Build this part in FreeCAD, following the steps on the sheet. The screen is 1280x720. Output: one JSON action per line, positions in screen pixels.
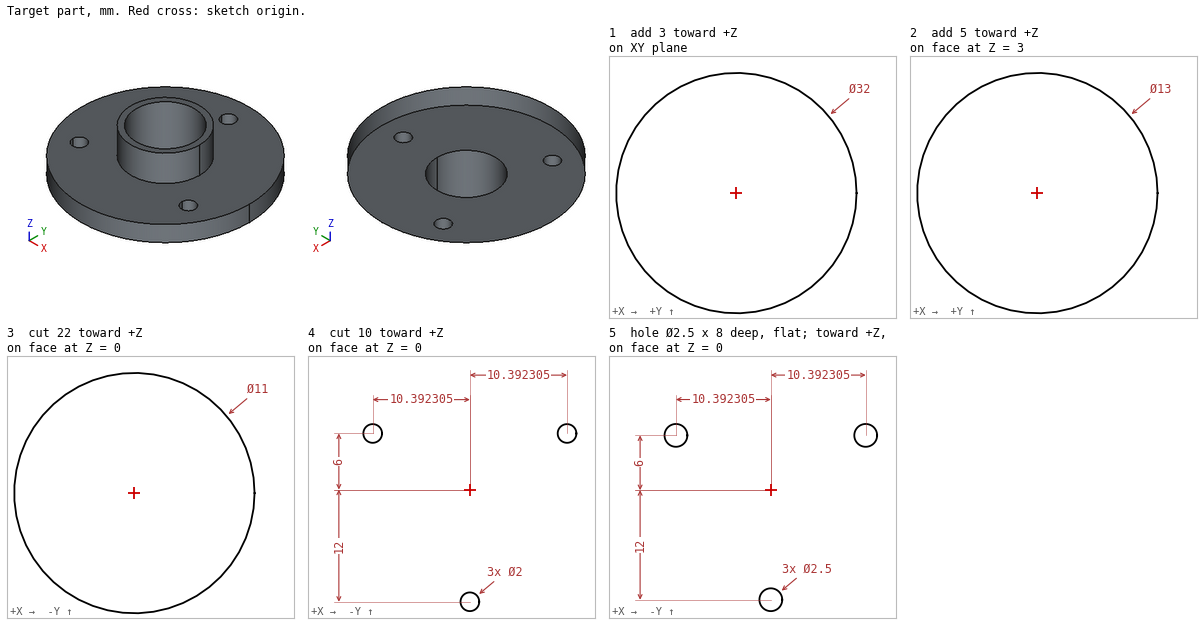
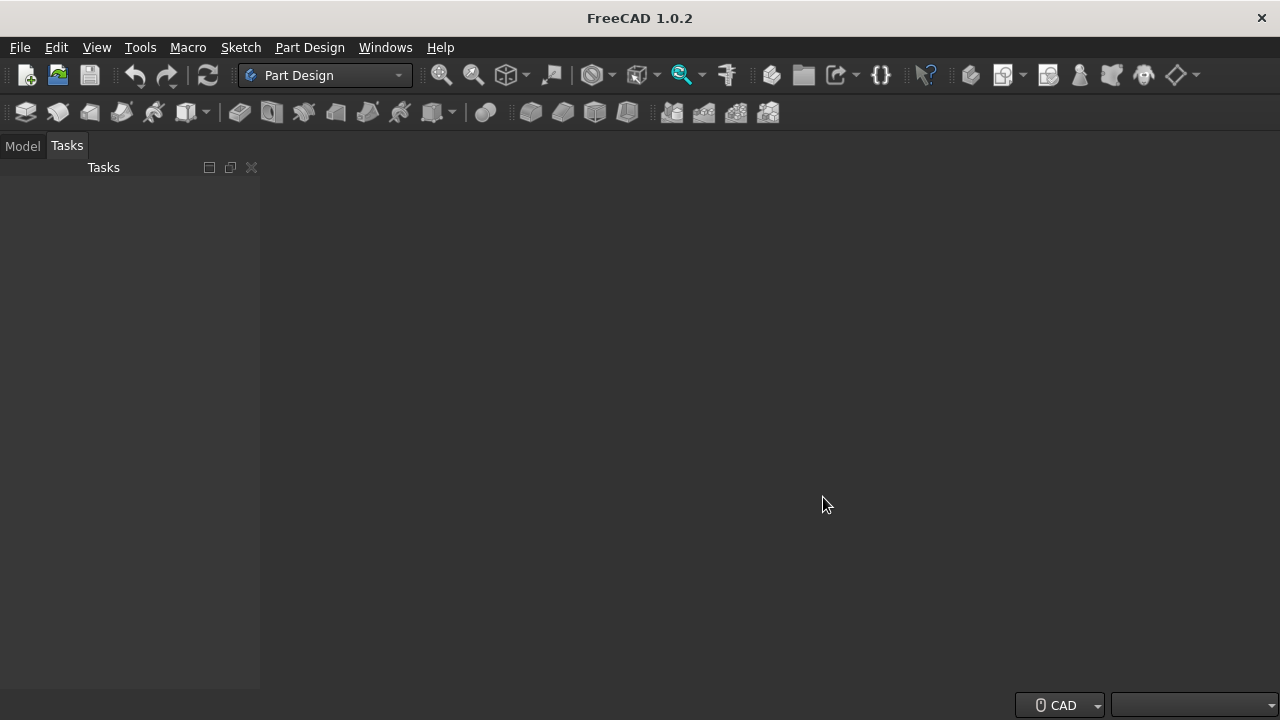
{"action": "left_click", "coordinate": [26, 76]}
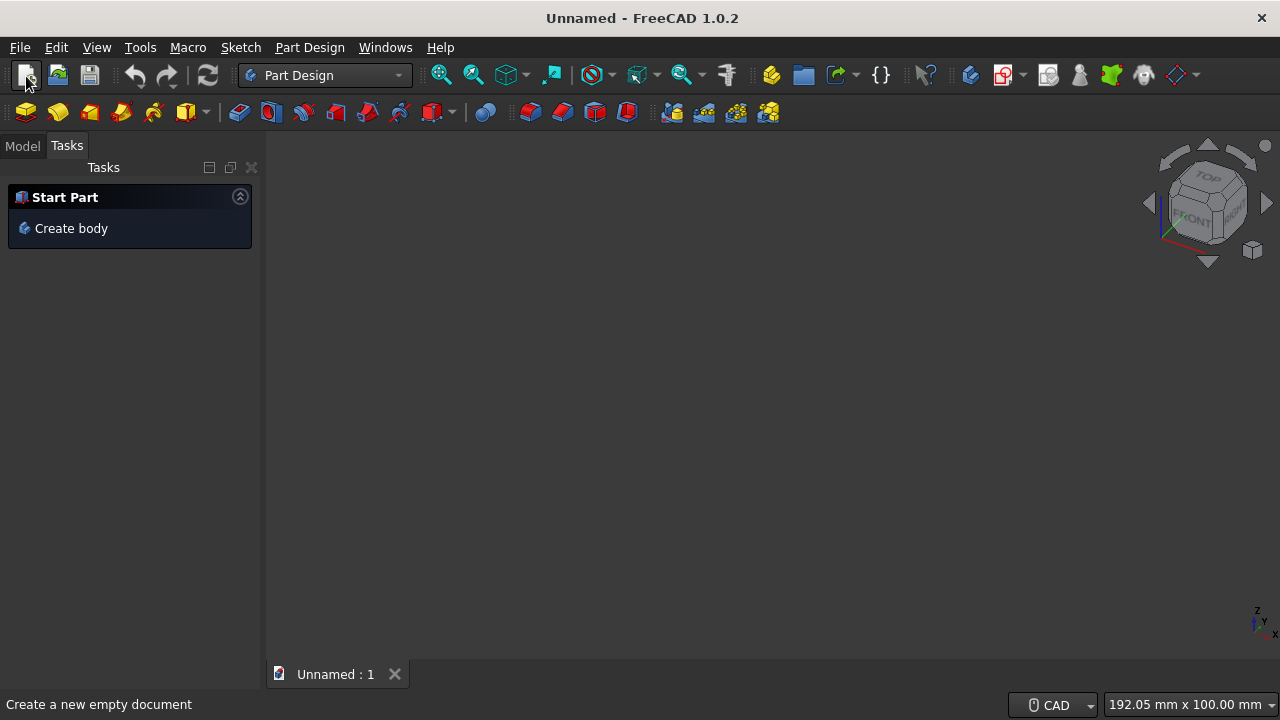
{"action": "left_click", "coordinate": [1004, 76]}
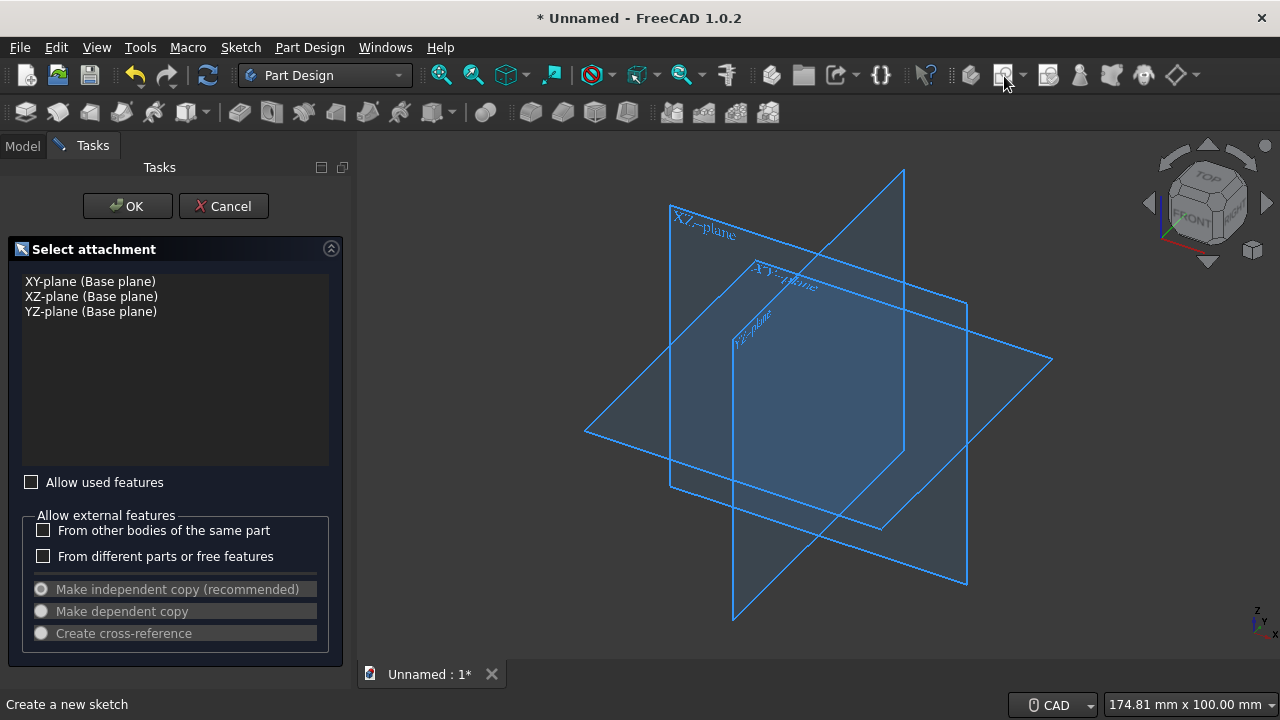
{"action": "left_click", "coordinate": [82, 282]}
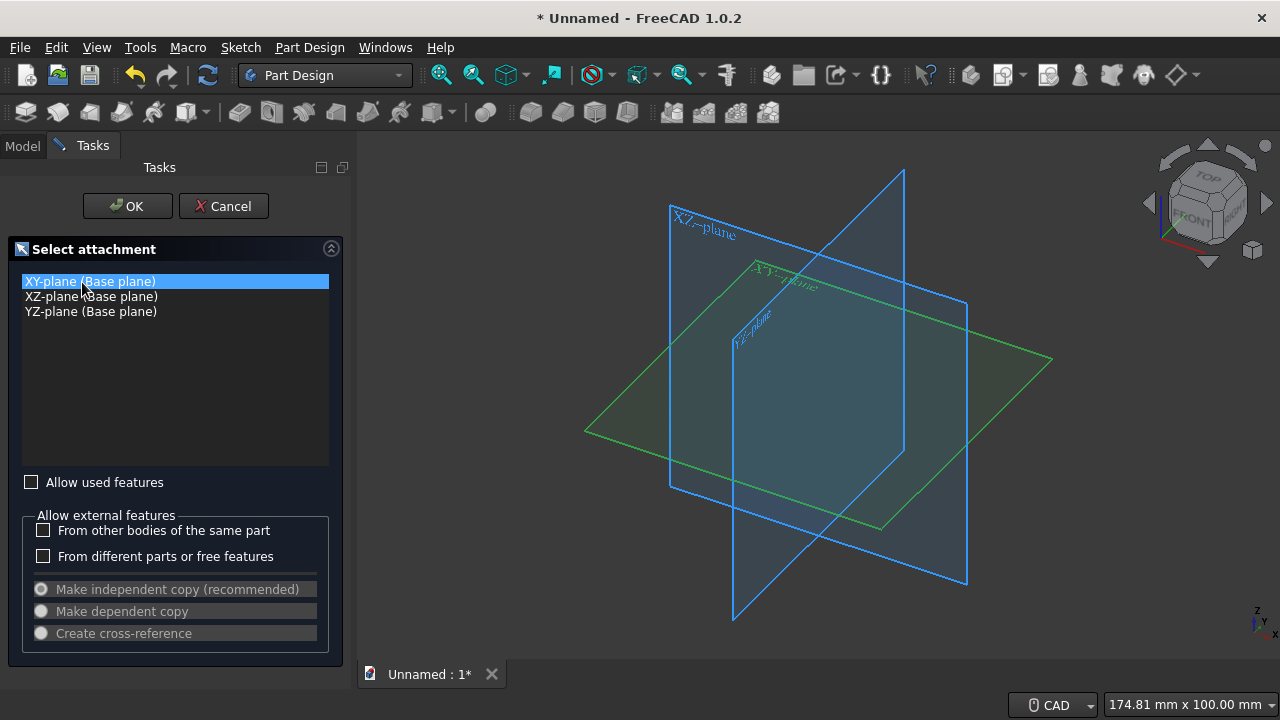
{"action": "left_click", "coordinate": [128, 206]}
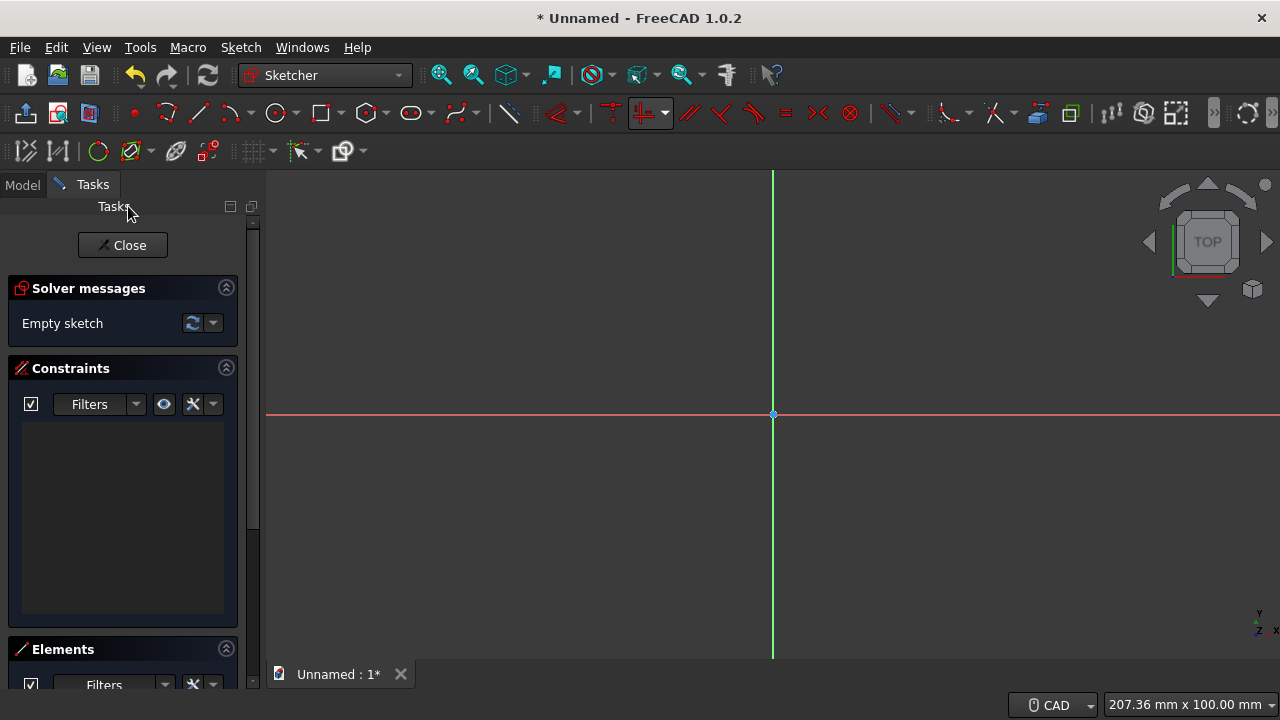
{"action": "scroll", "coordinate": [856, 415], "scroll_direction": "up", "scroll_amount": 3}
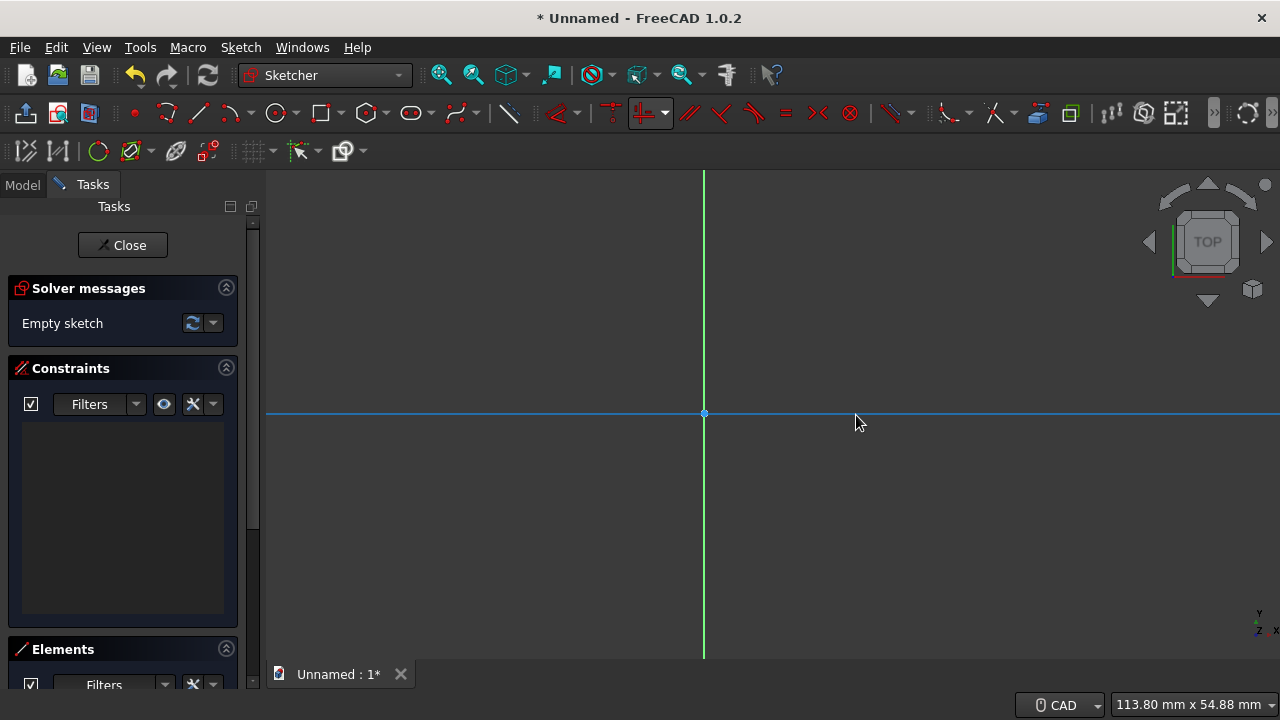
{"action": "left_click", "coordinate": [276, 114]}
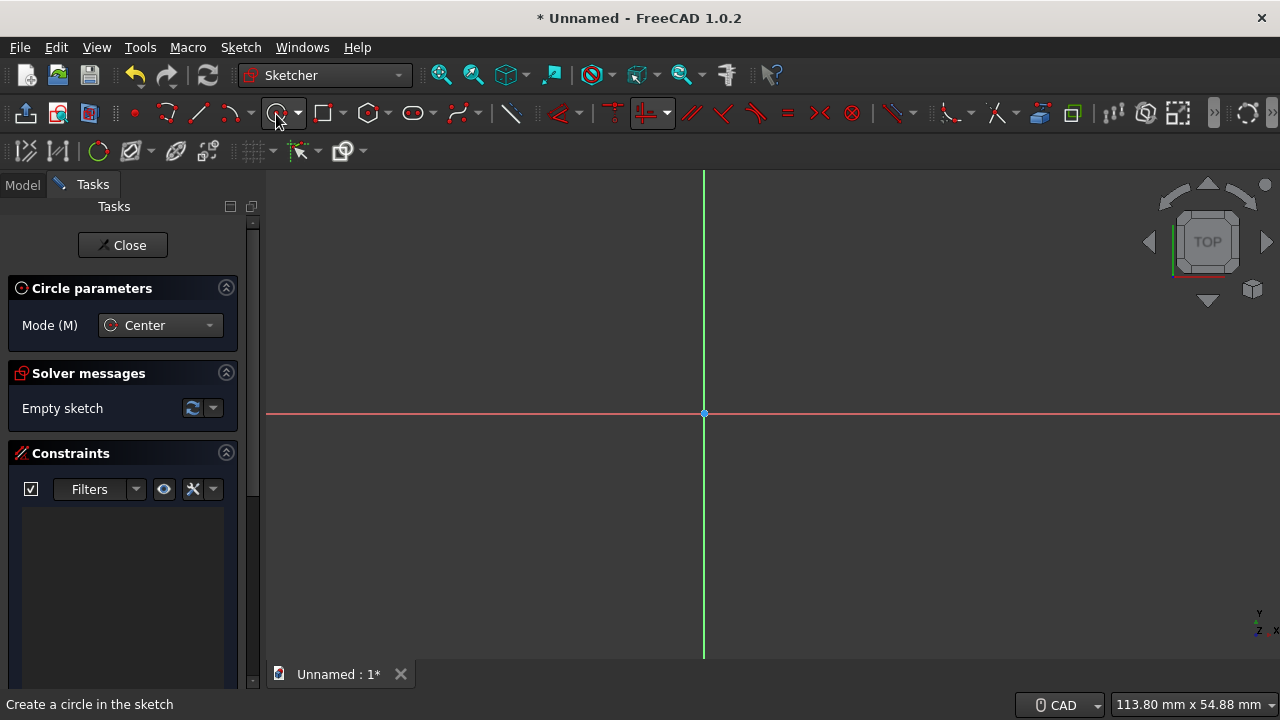
{"action": "left_click", "coordinate": [704, 414]}
{"action": "mouse_move", "coordinate": [805, 313]}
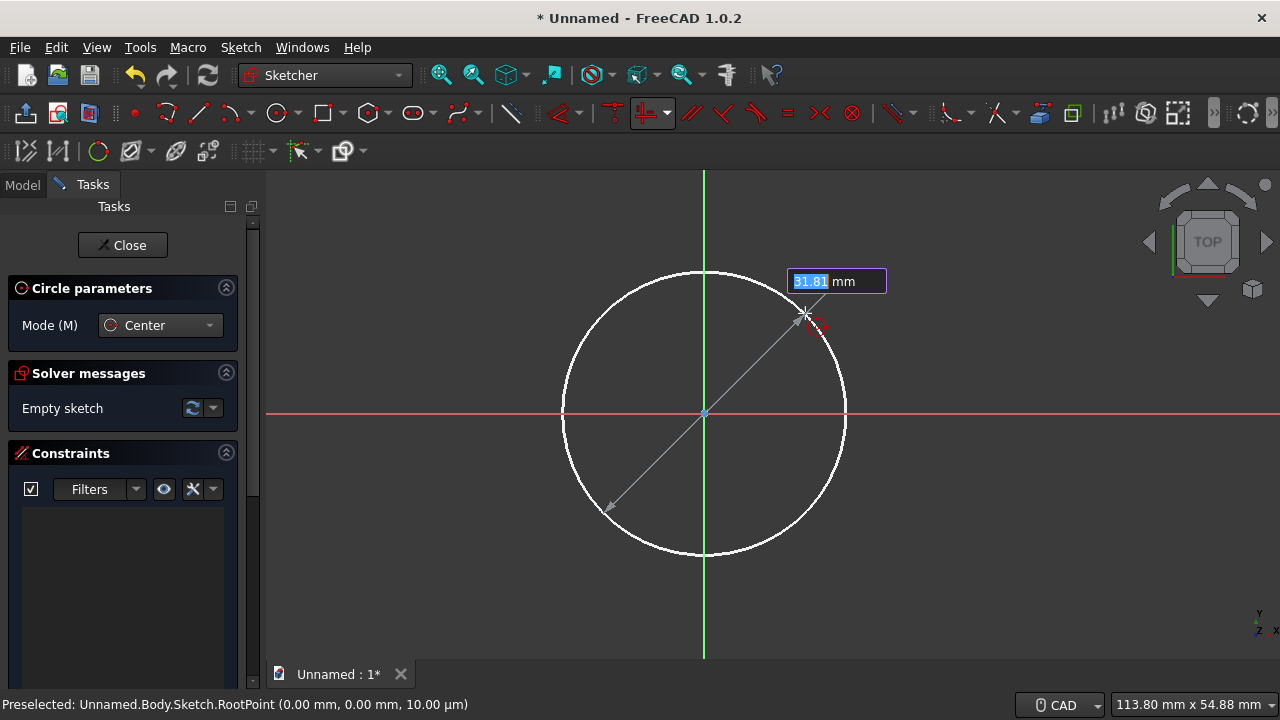
{"action": "type", "text": "32"}
{"action": "key", "text": "Return"}
{"action": "key", "text": "Escape"}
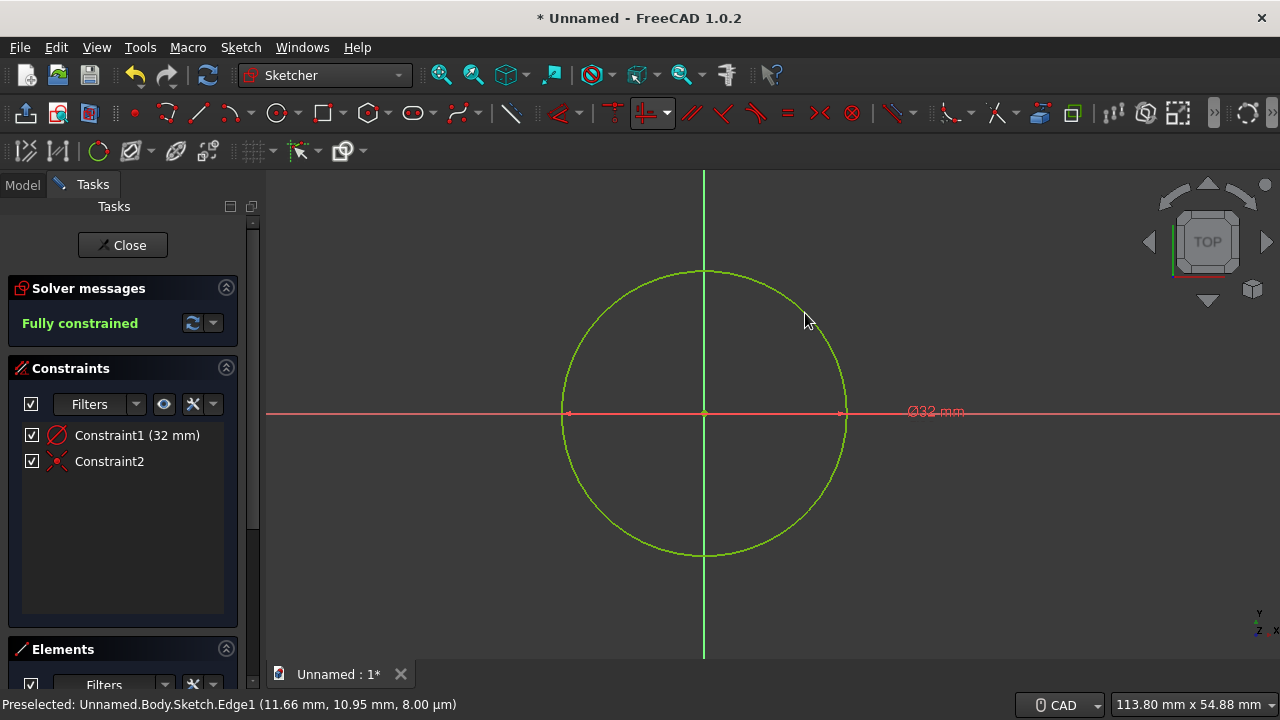
{"action": "left_click", "coordinate": [123, 245]}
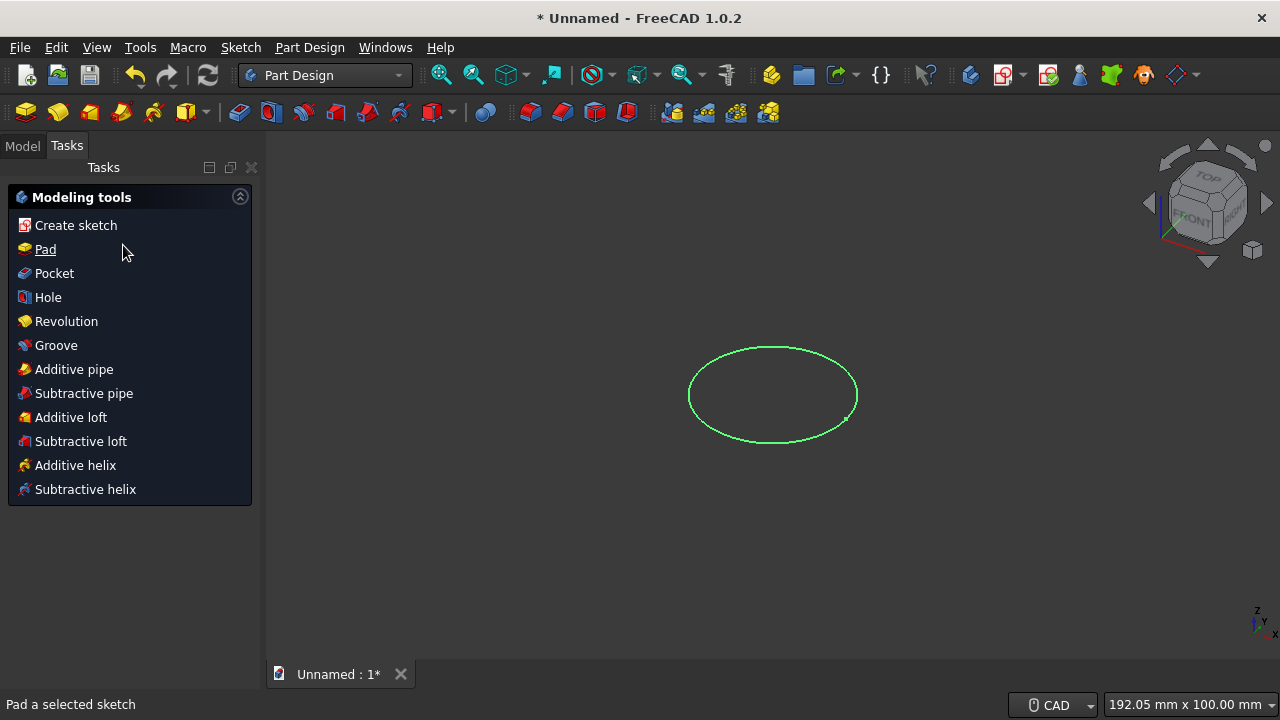
{"action": "left_click", "coordinate": [26, 112]}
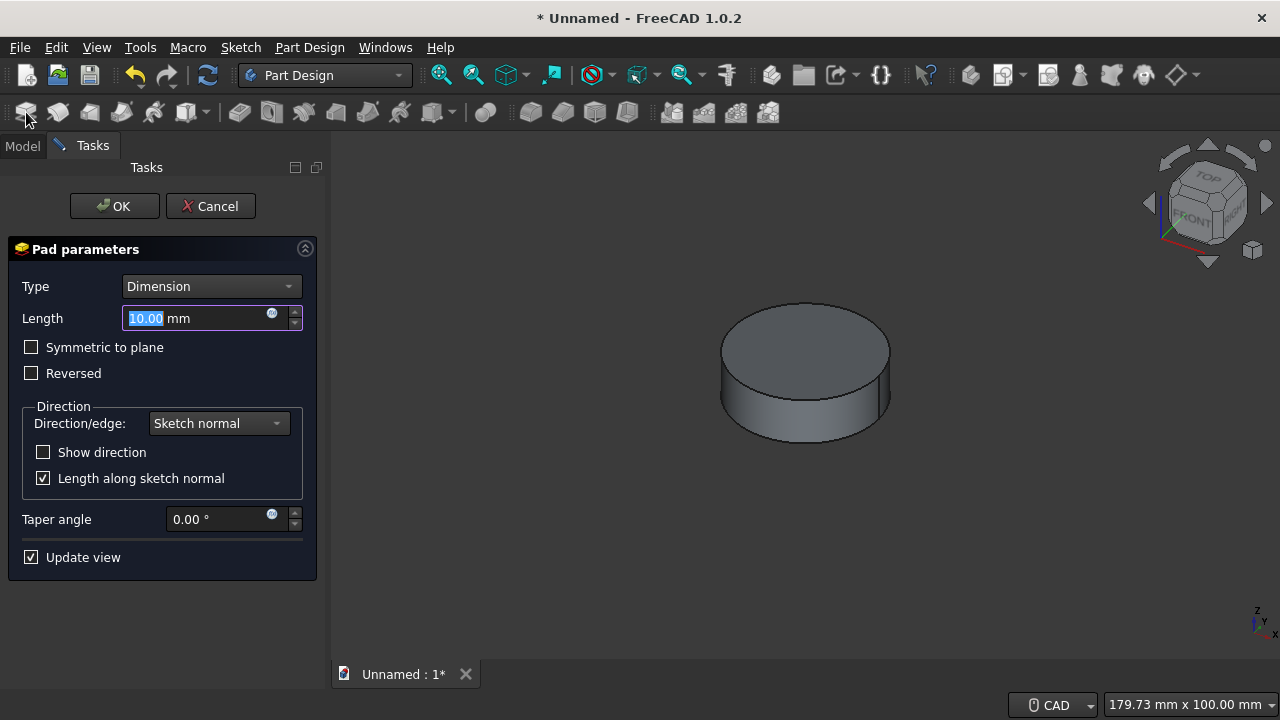
{"action": "type", "text": "3"}
{"action": "key", "text": "Tab"}